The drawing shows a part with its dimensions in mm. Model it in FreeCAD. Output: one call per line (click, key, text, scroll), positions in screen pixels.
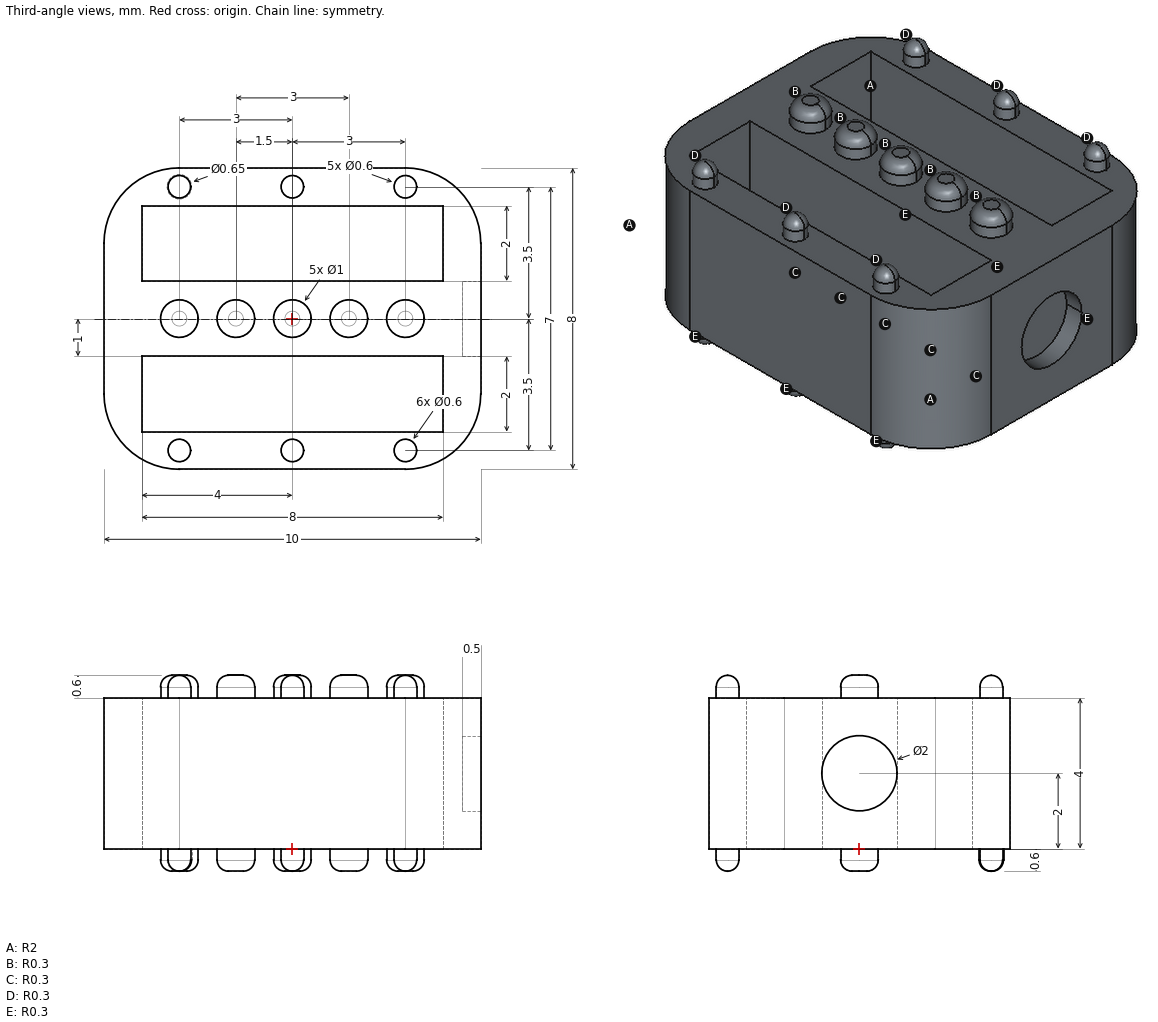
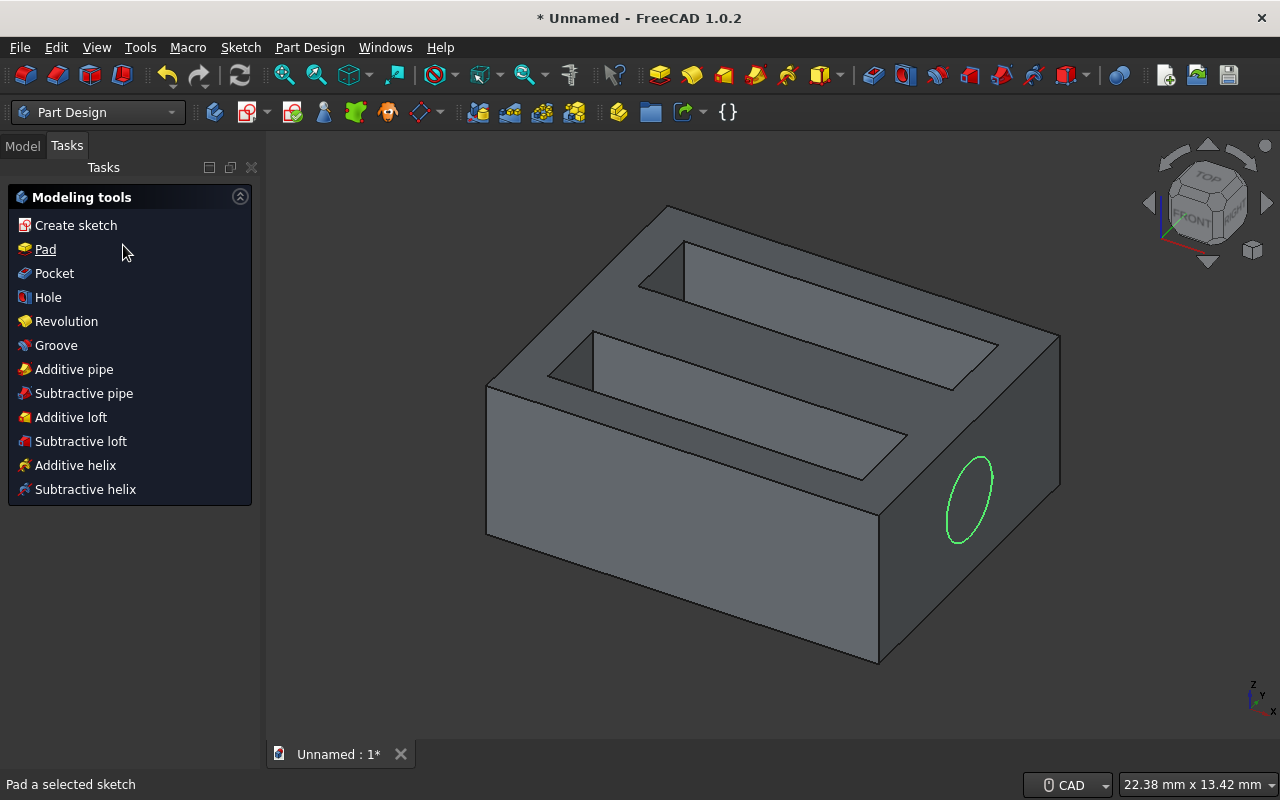
click(874, 76)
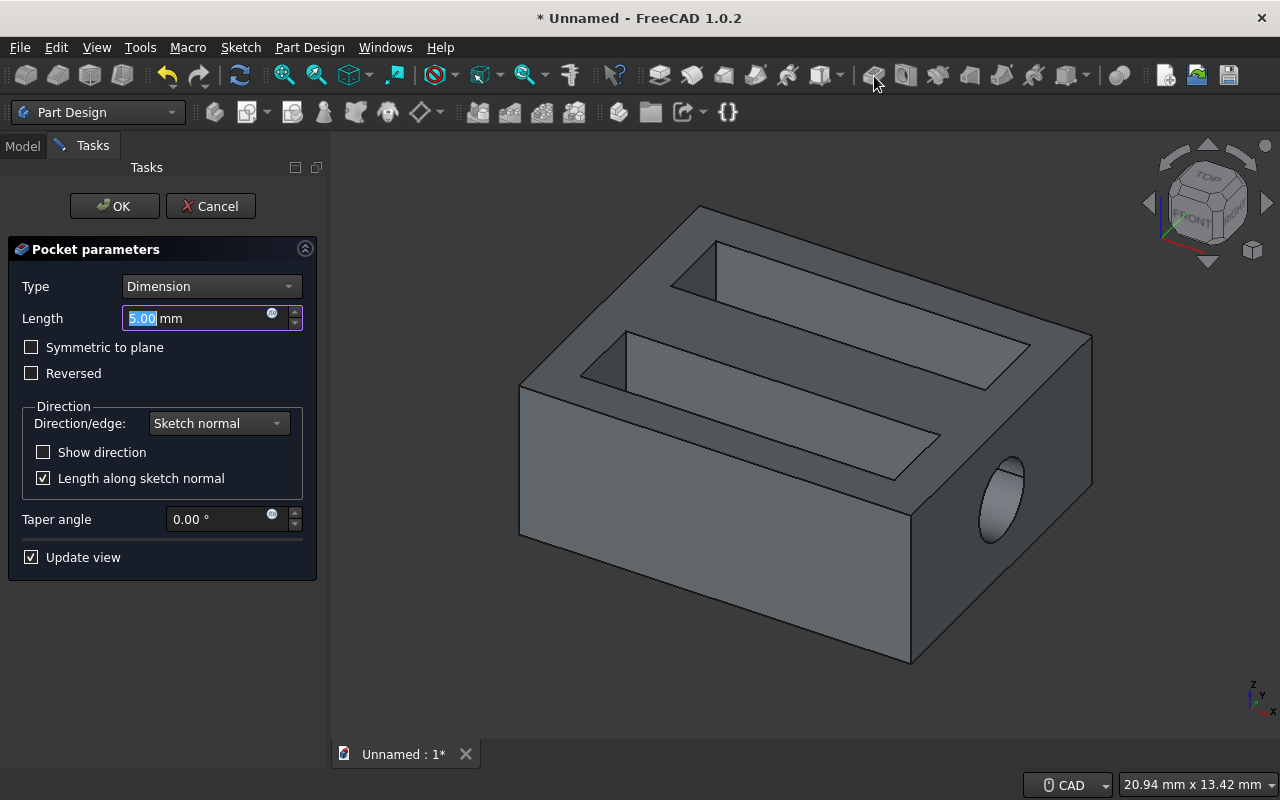
text(0.5)
key(Tab)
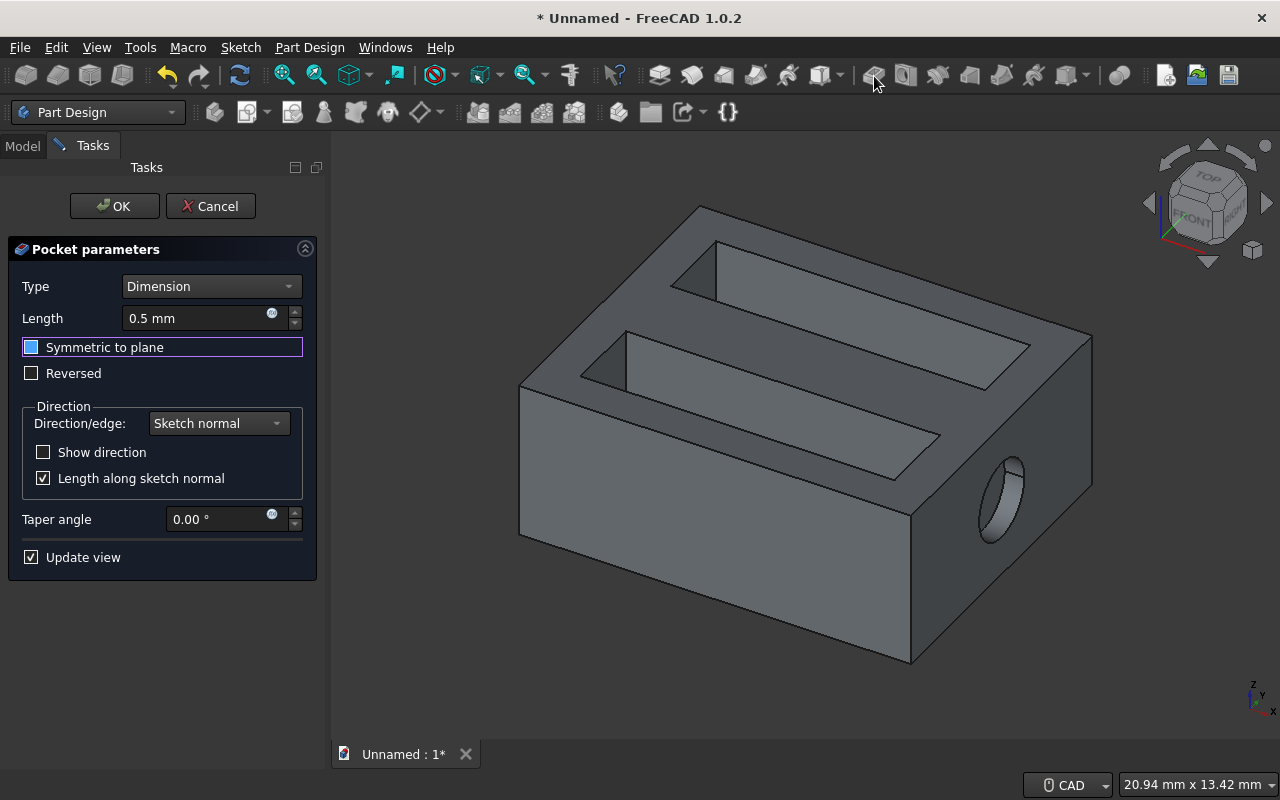
click(115, 206)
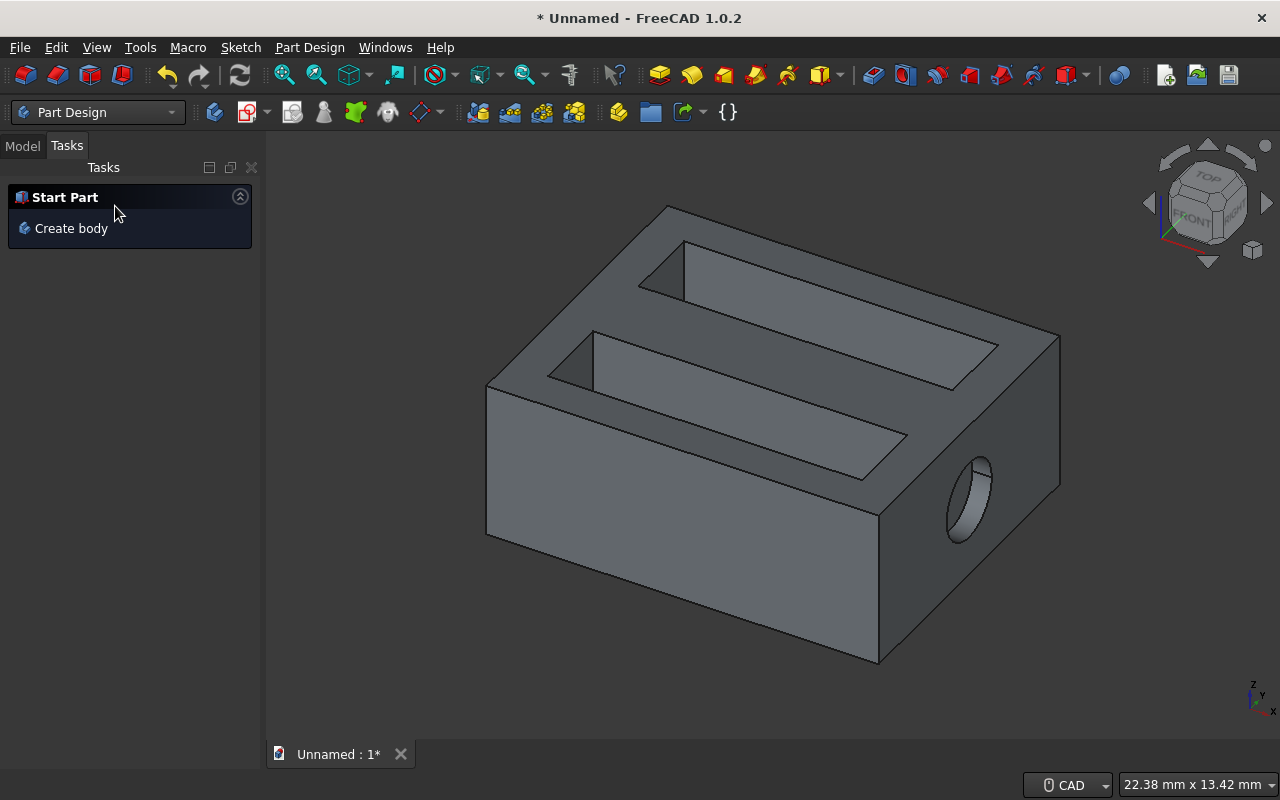
click(879, 589)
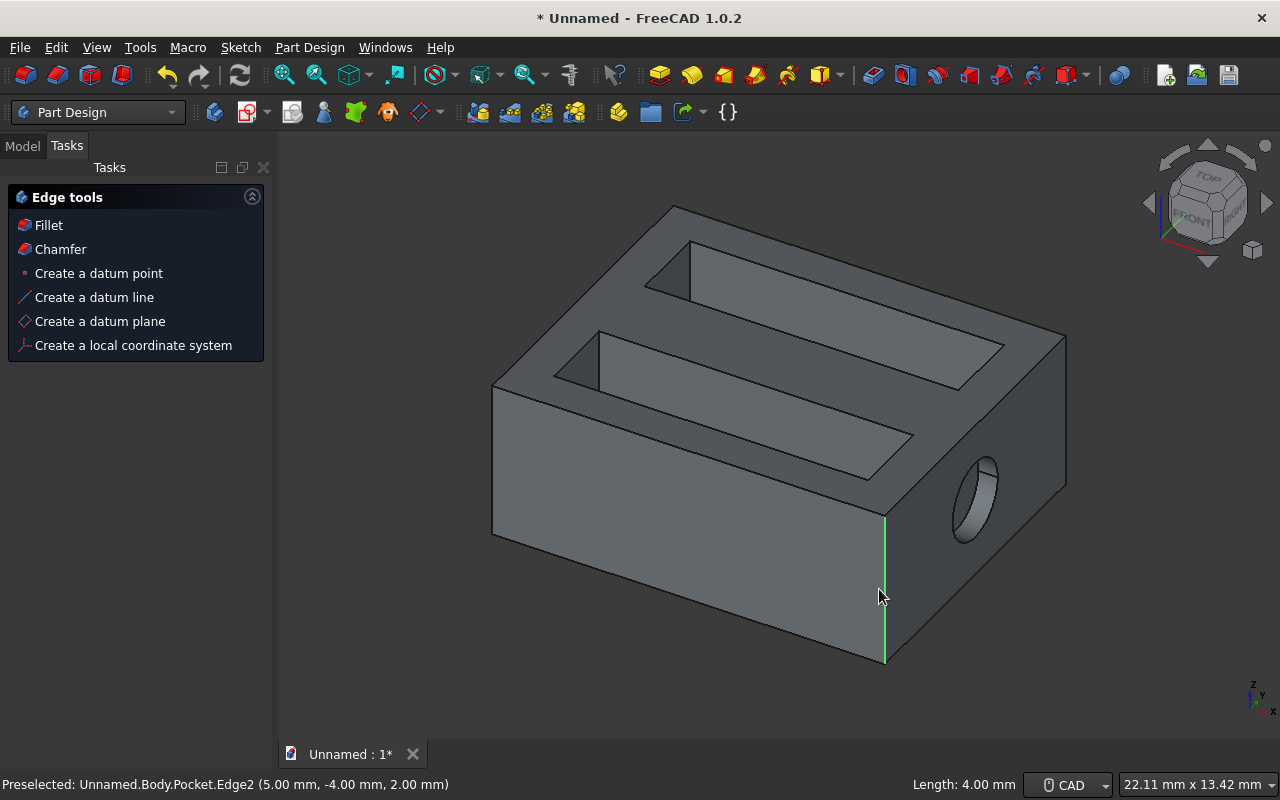
key(0)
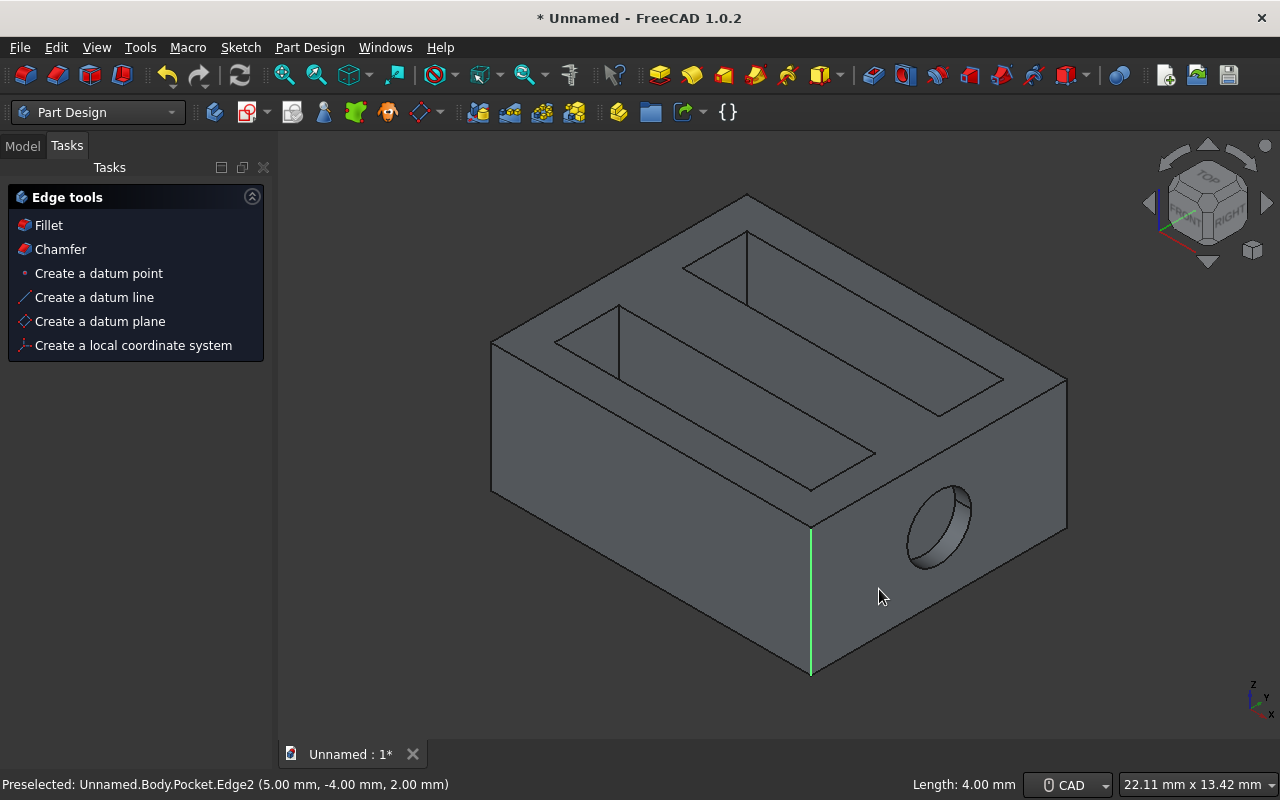
key(2)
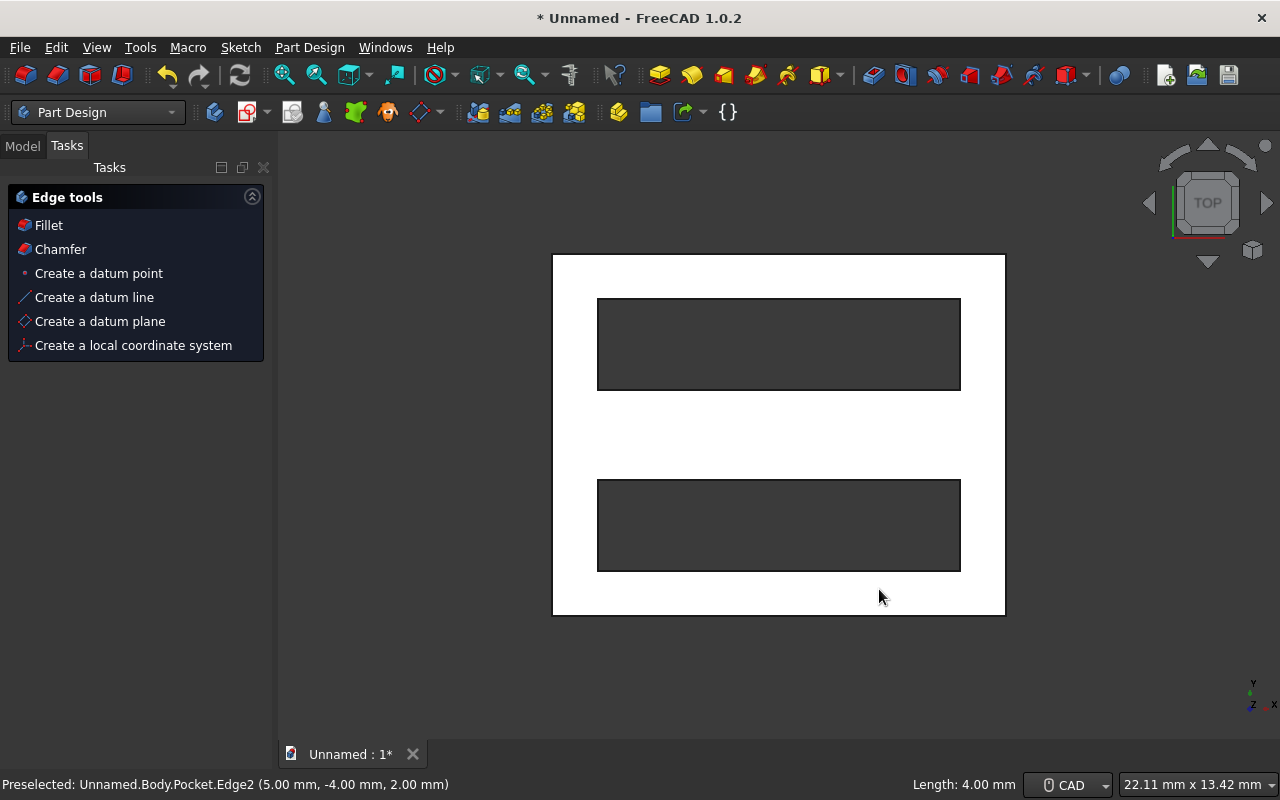
key(1)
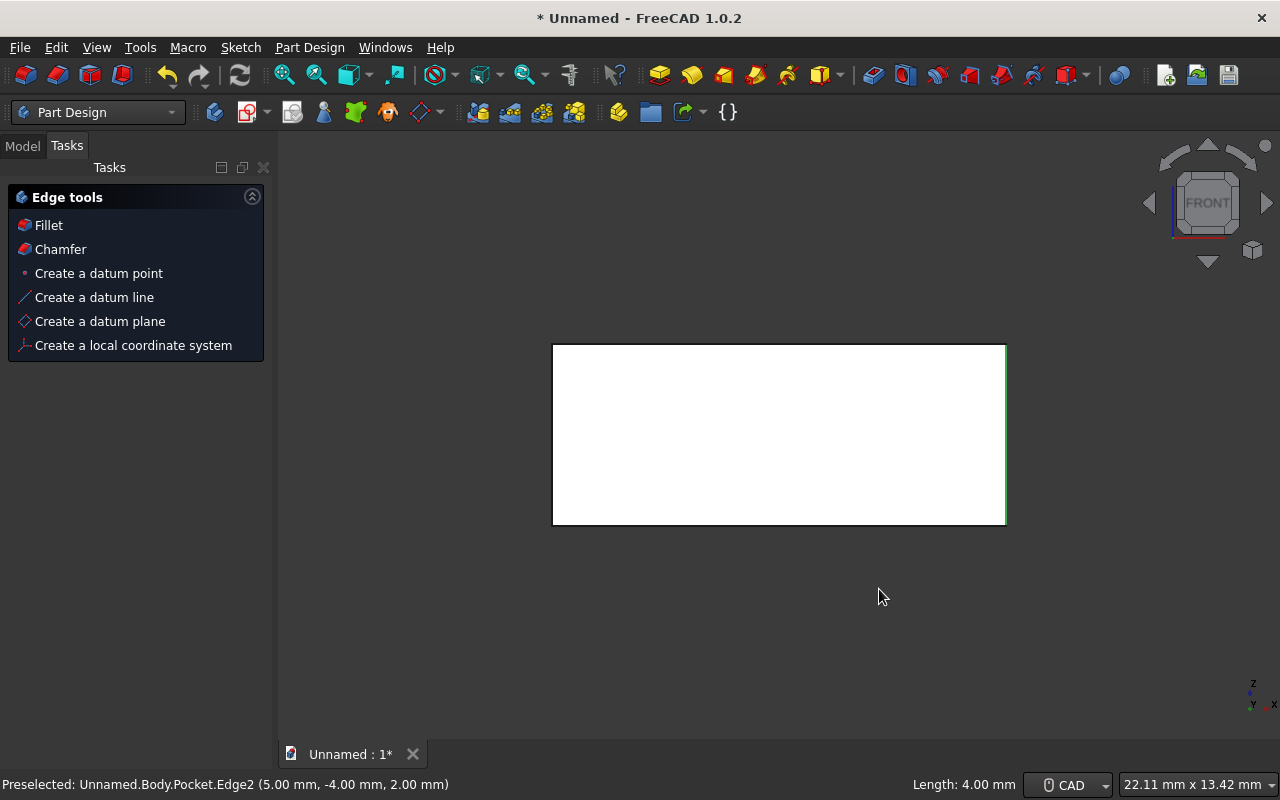
click(552, 434, ctrl)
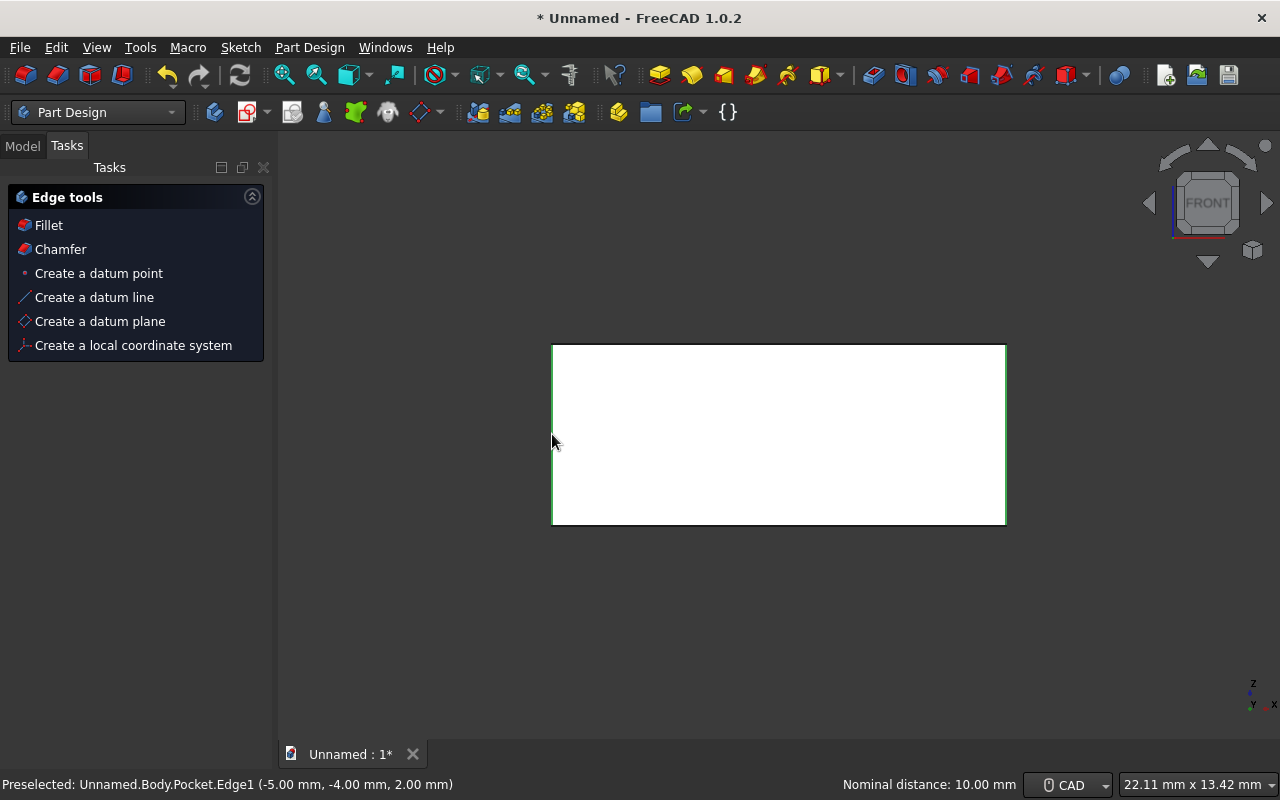
key(3)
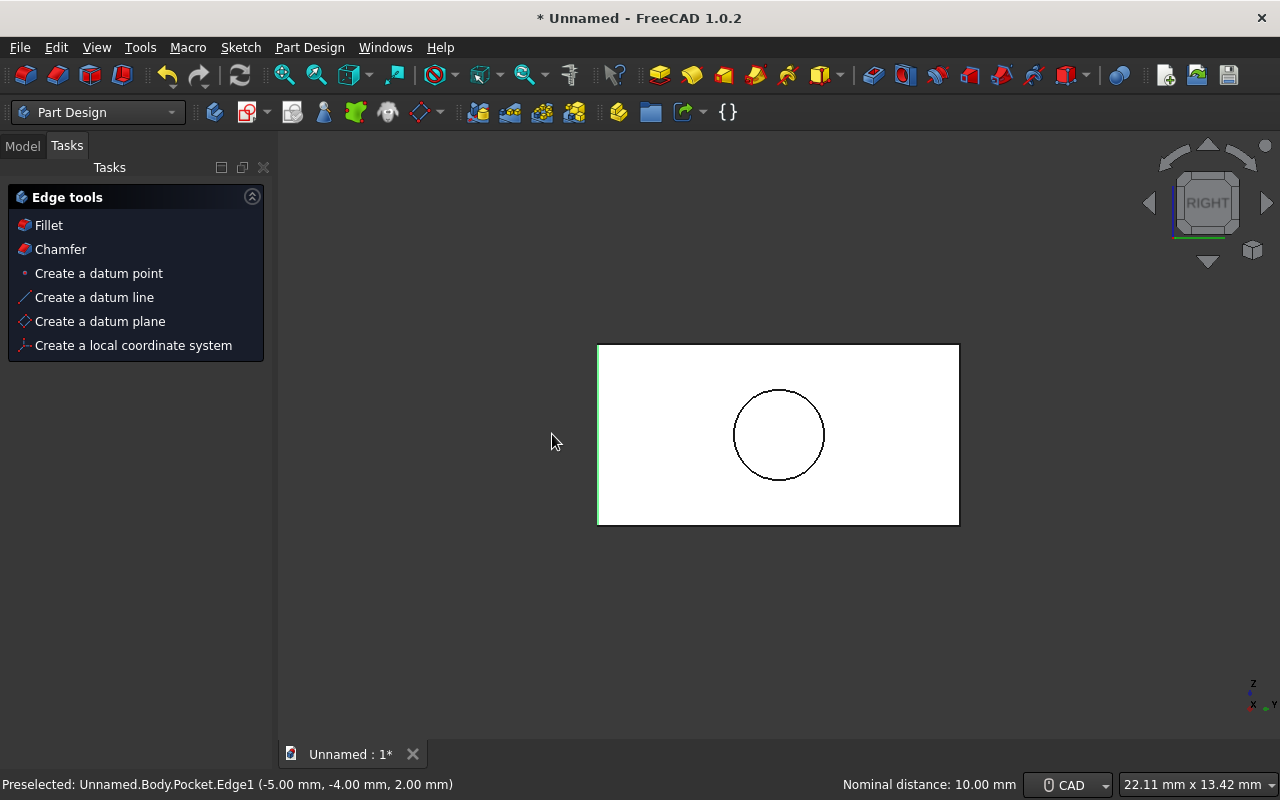
click(286, 76)